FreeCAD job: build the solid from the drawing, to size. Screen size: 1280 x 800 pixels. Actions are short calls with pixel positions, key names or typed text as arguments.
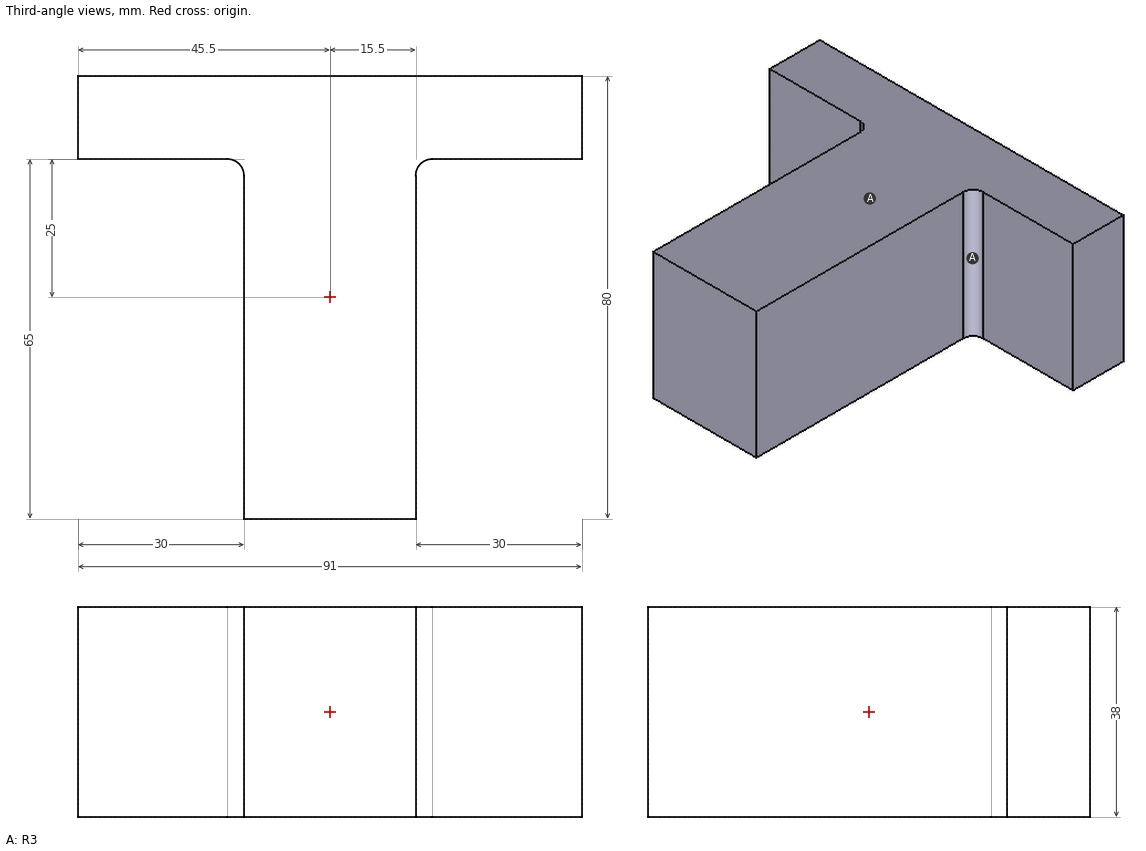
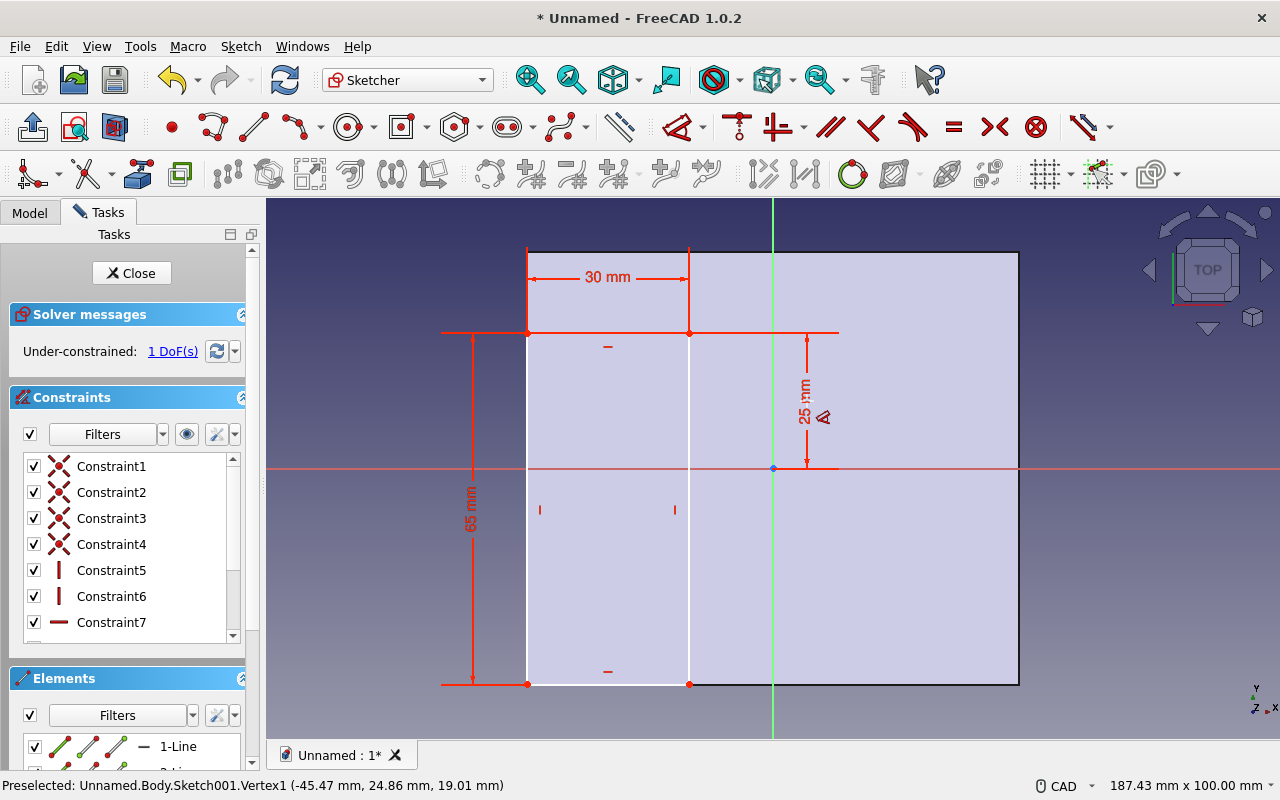
click(527, 333)
click(650, 299)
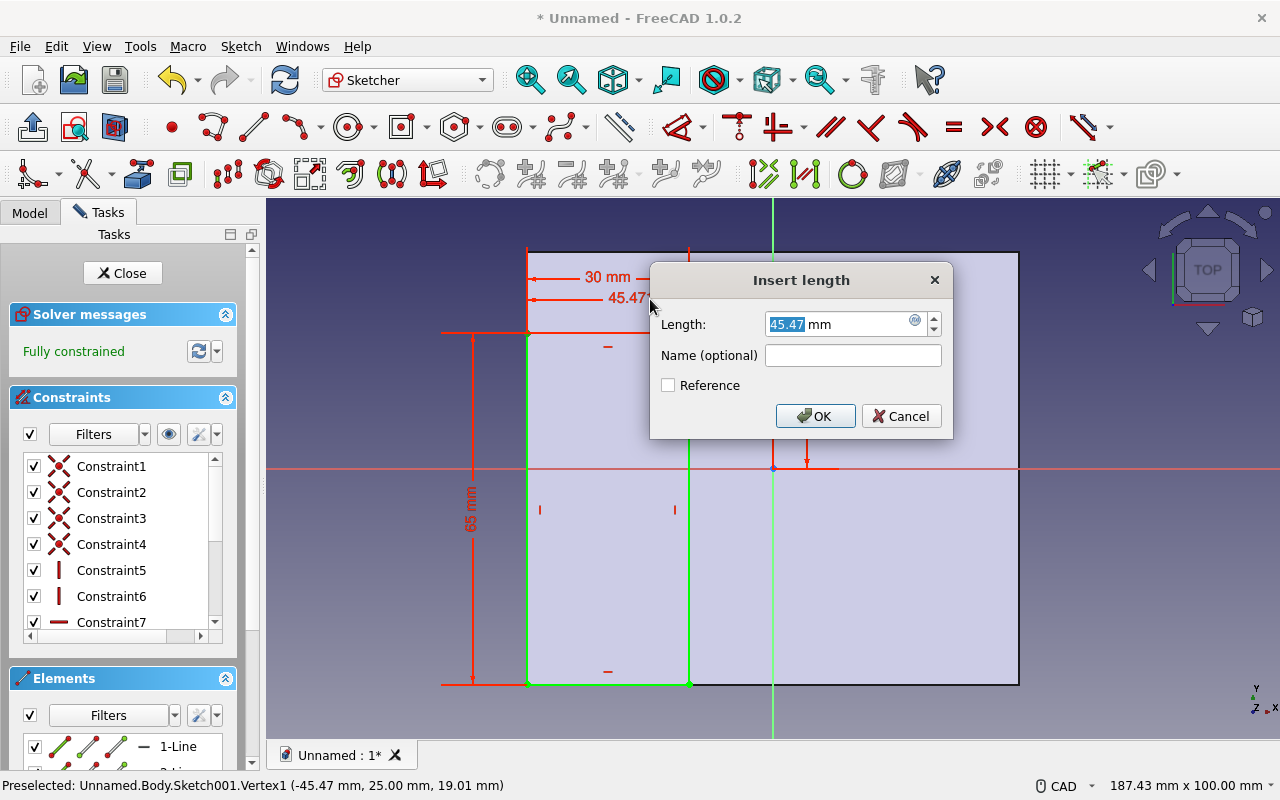
text(45.5)
key(Return)
key(Escape)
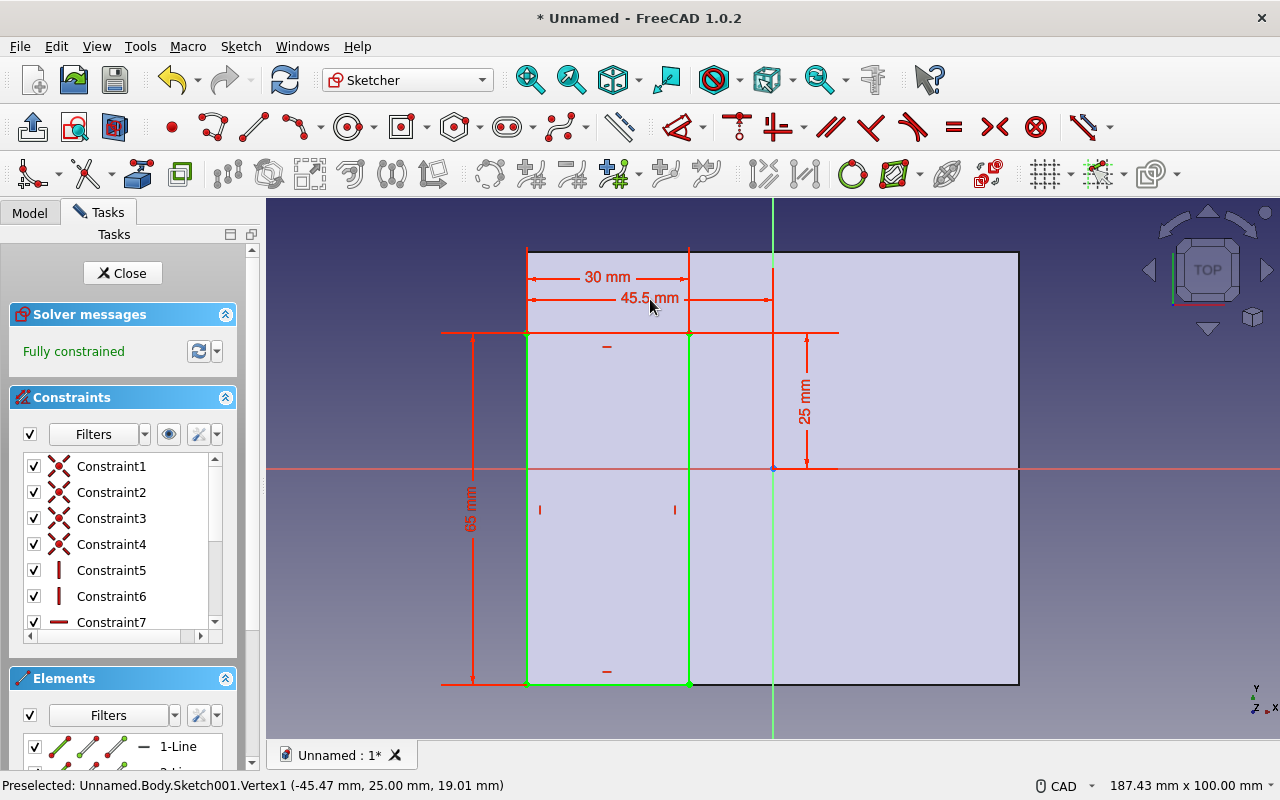
click(123, 273)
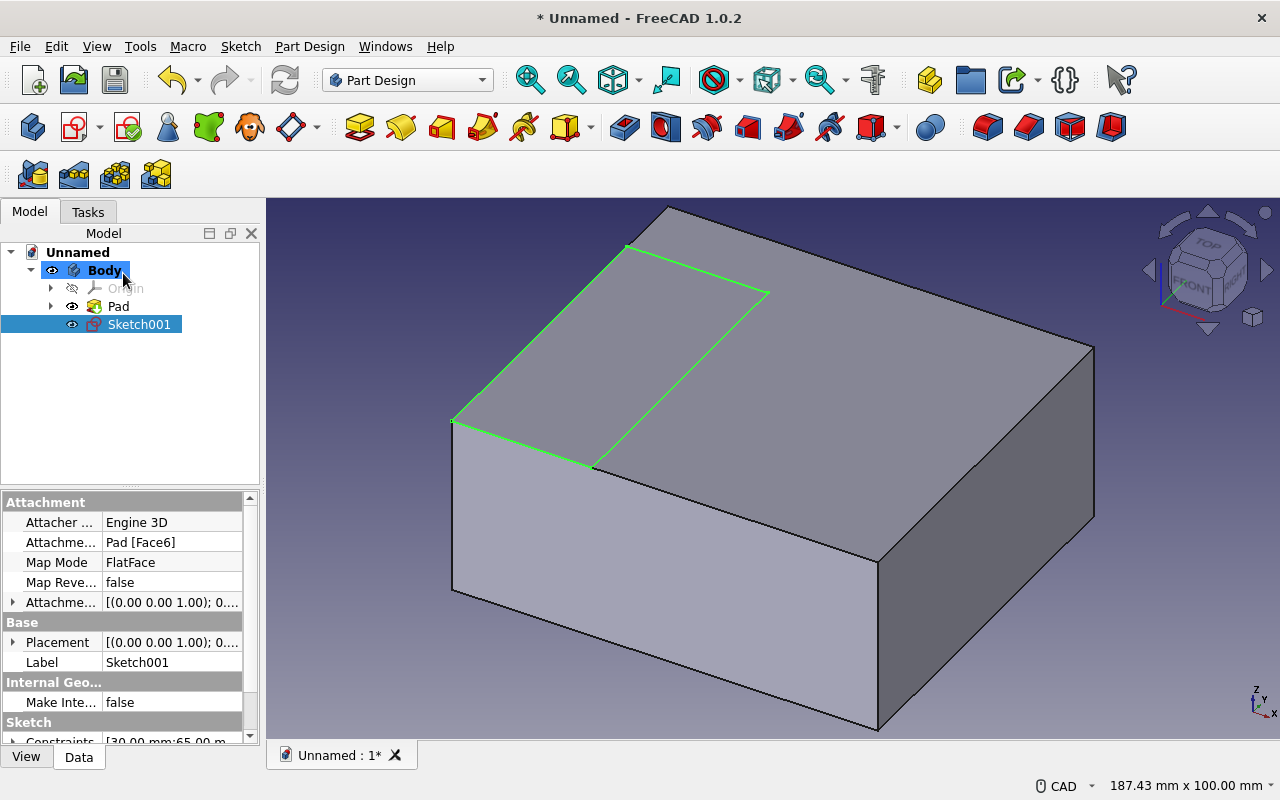
click(625, 128)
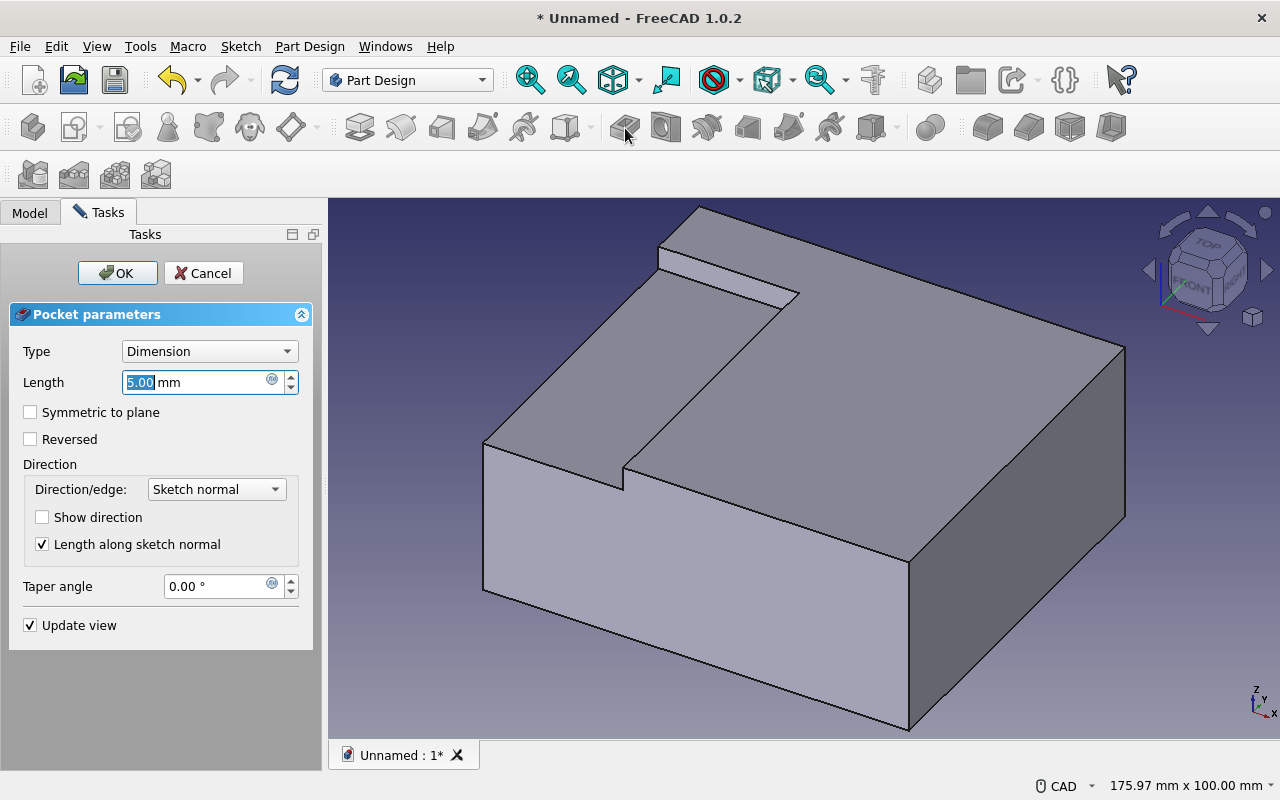
click(210, 352)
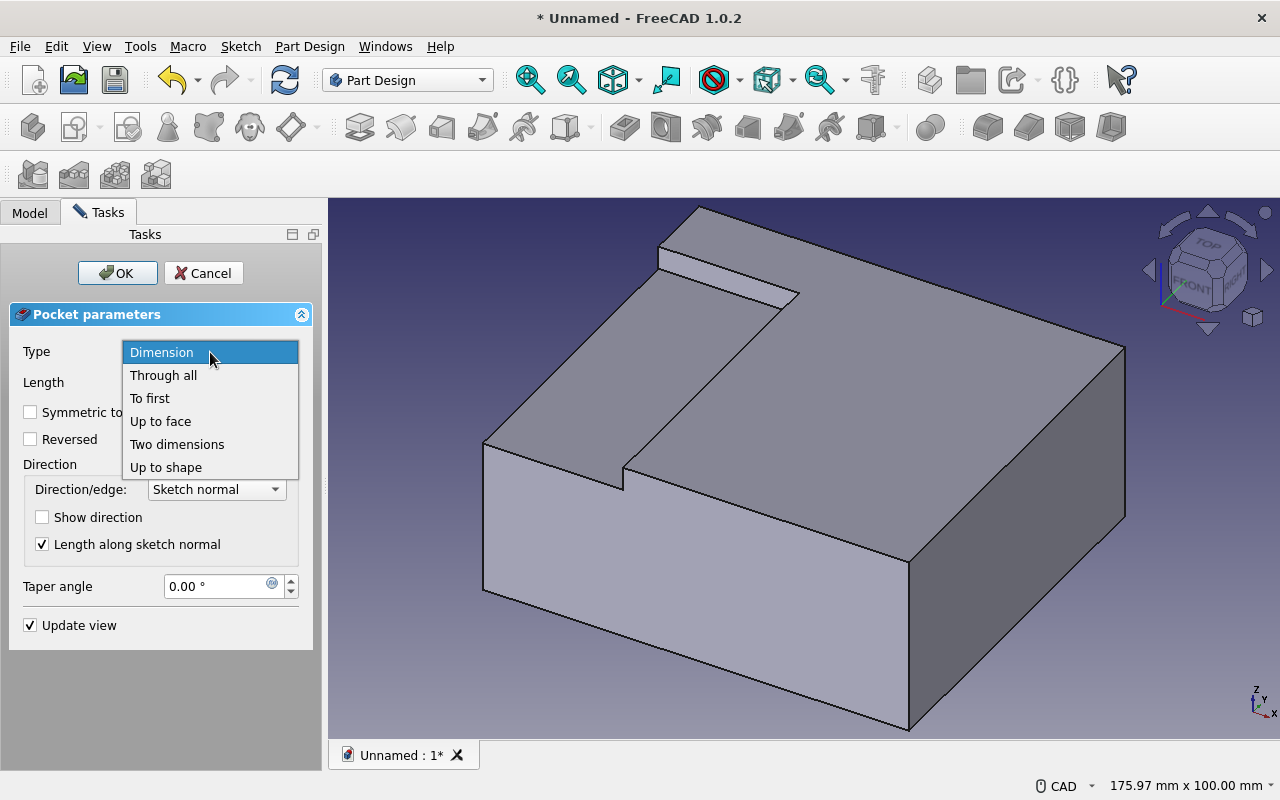
click(208, 398)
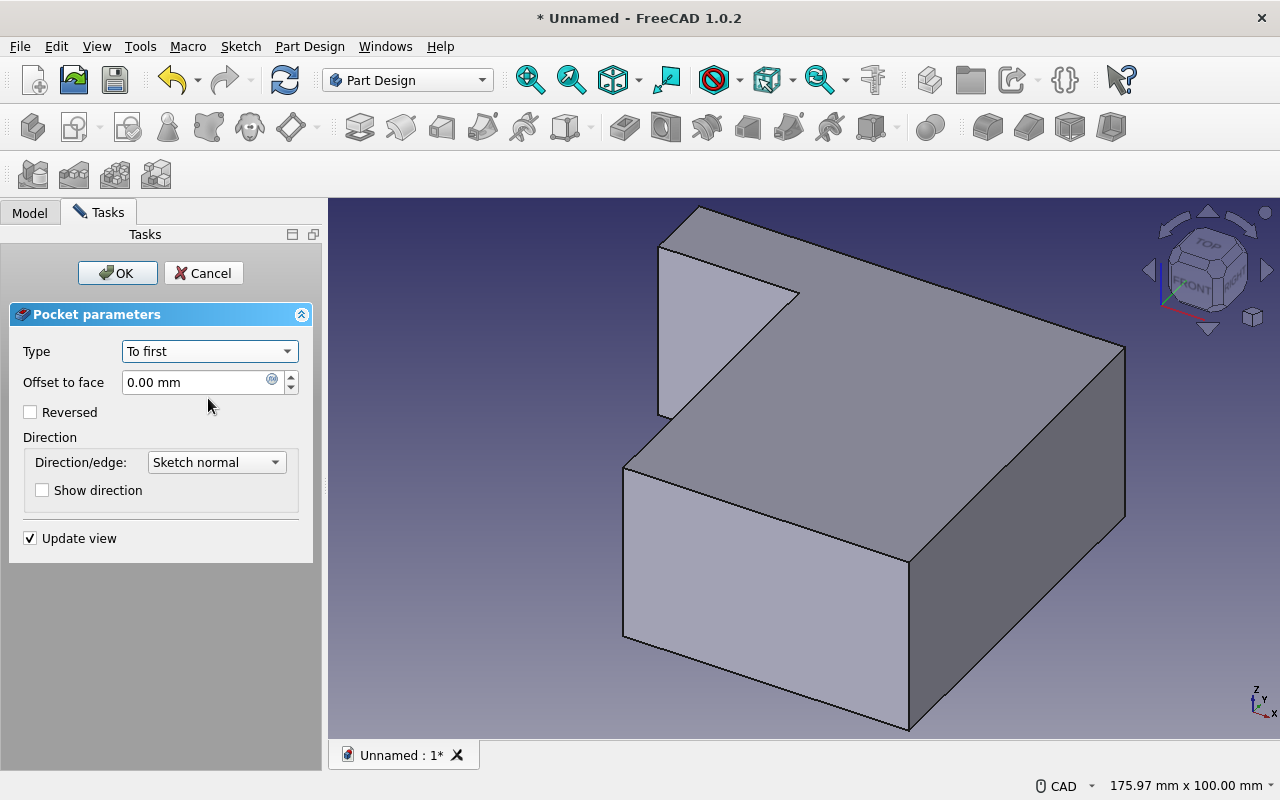
click(118, 273)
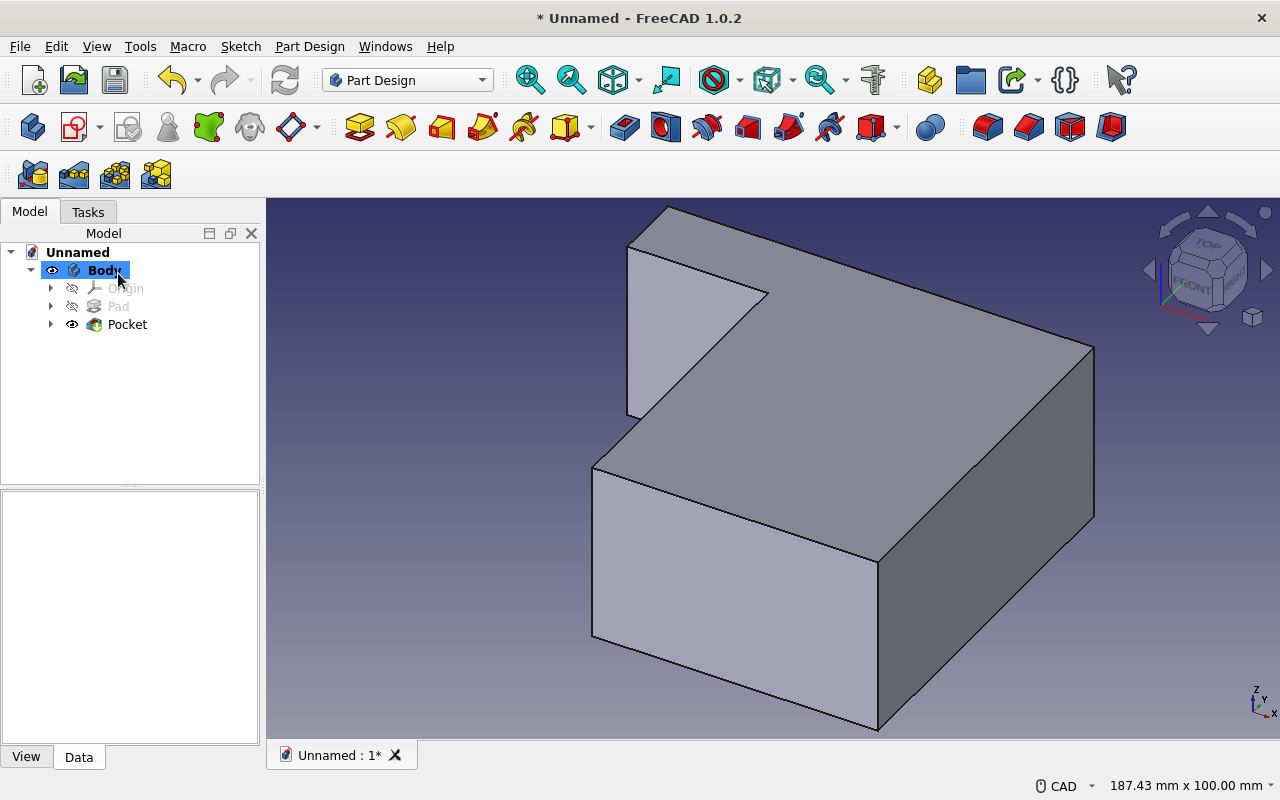
click(865, 373)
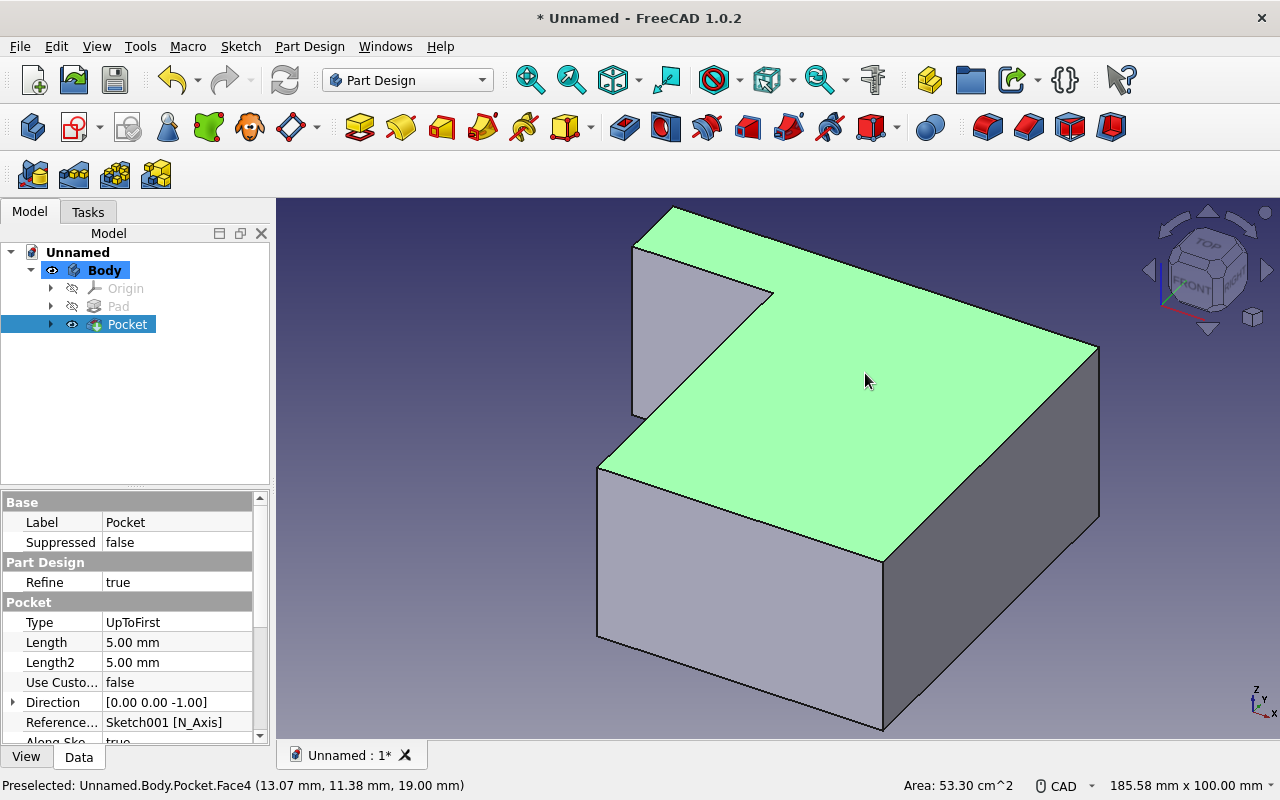
click(74, 128)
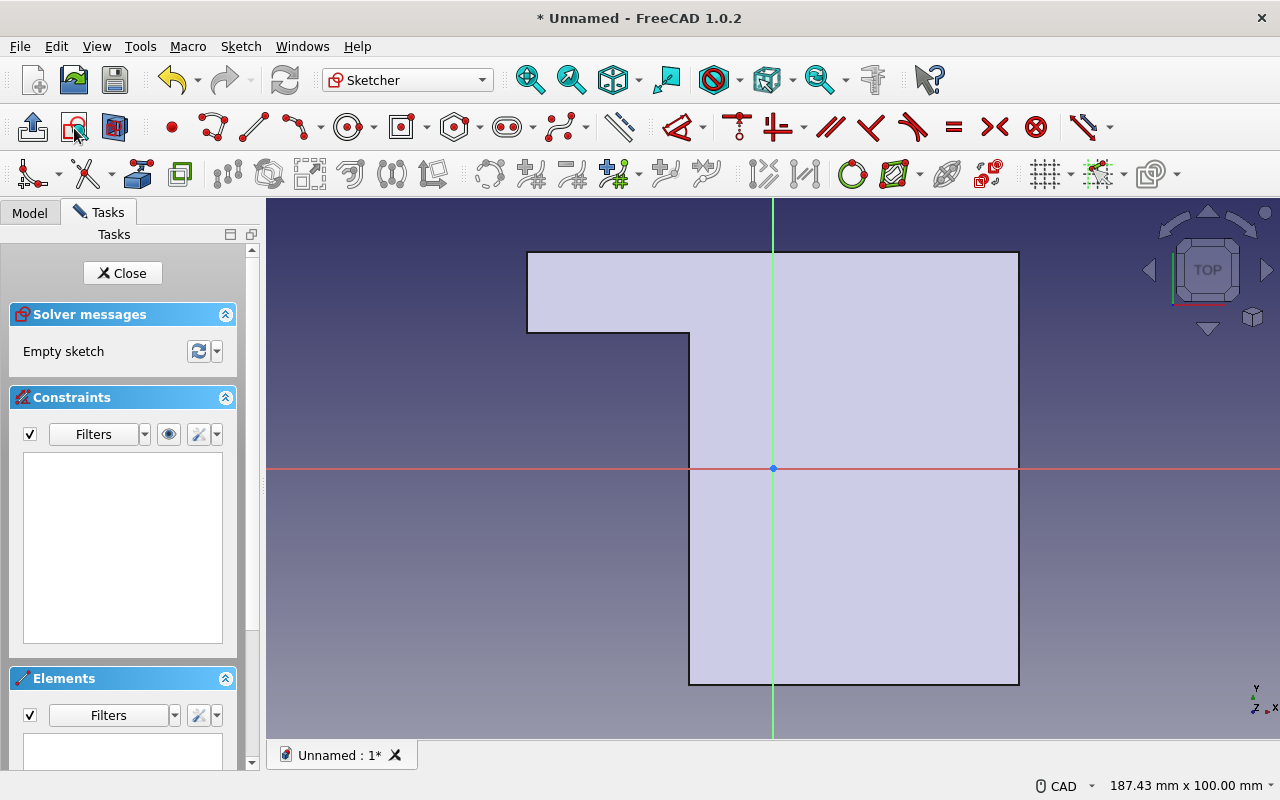
key(g)
key(r)